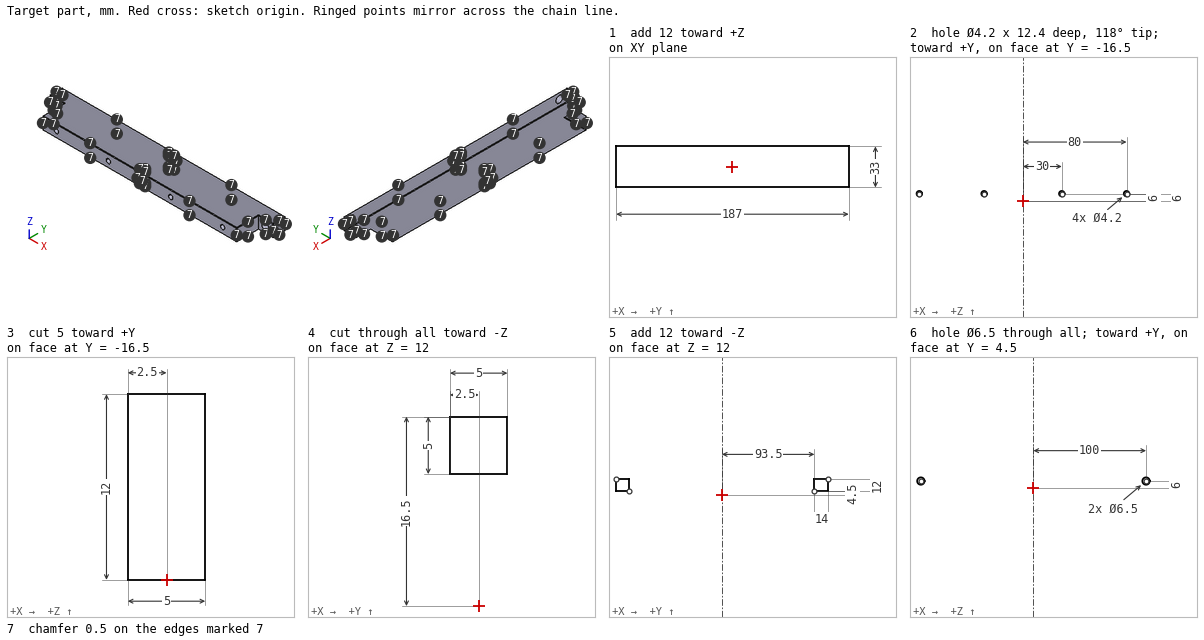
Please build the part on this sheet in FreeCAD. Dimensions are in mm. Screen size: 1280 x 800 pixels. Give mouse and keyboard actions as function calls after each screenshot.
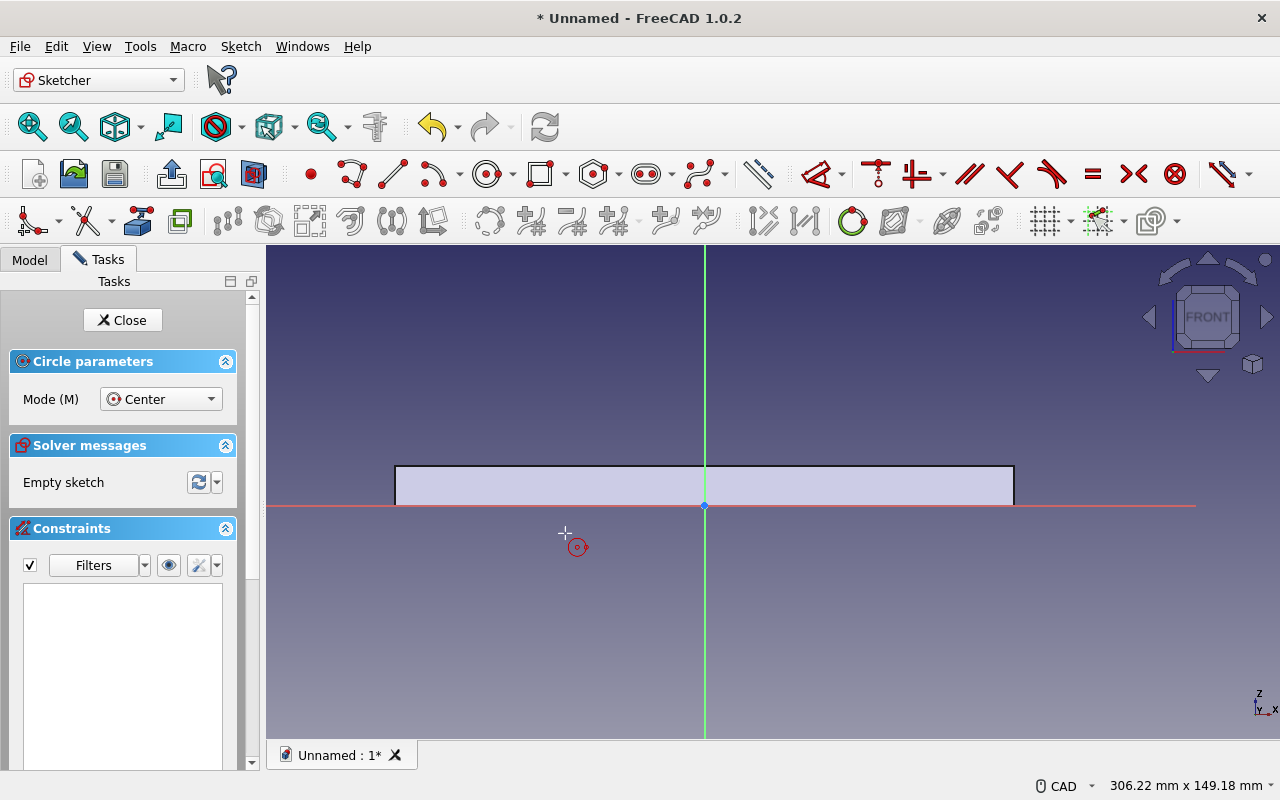
scroll(969, 486, up, 6)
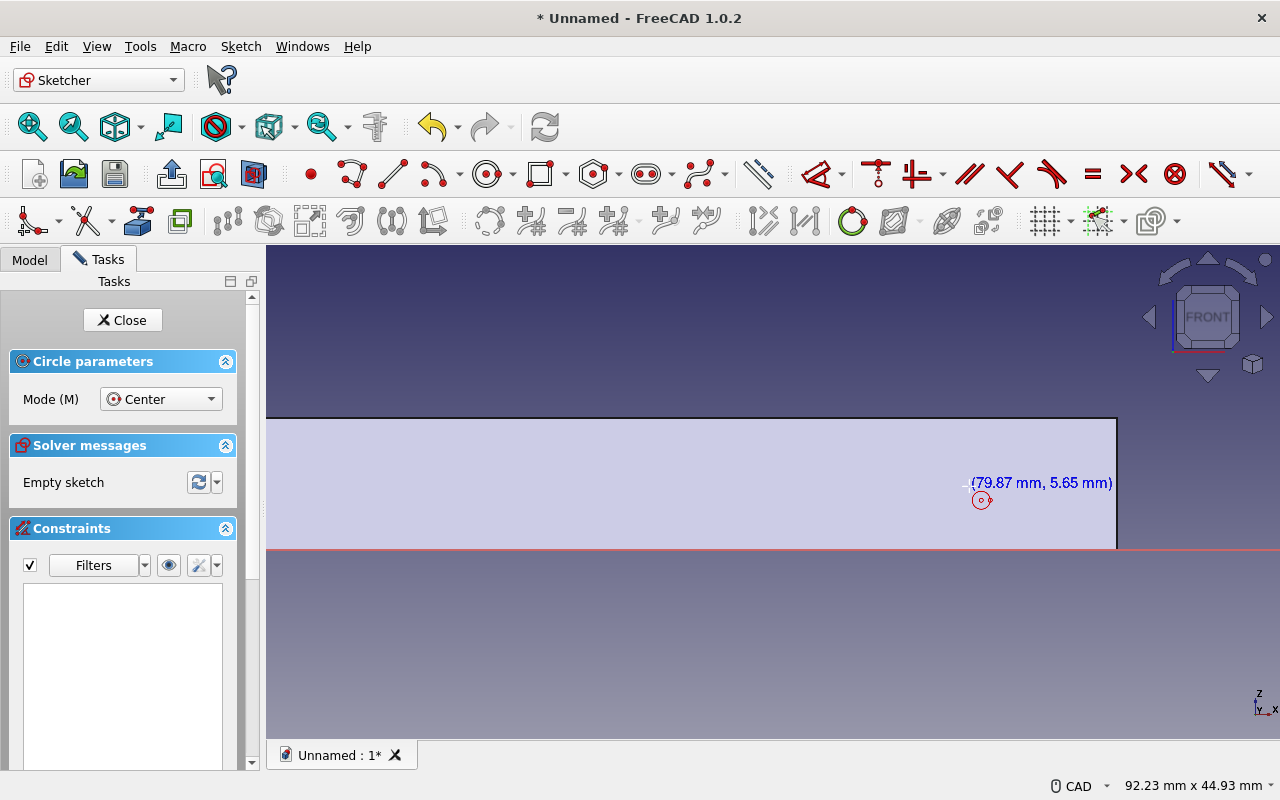
click(969, 484)
click(985, 468)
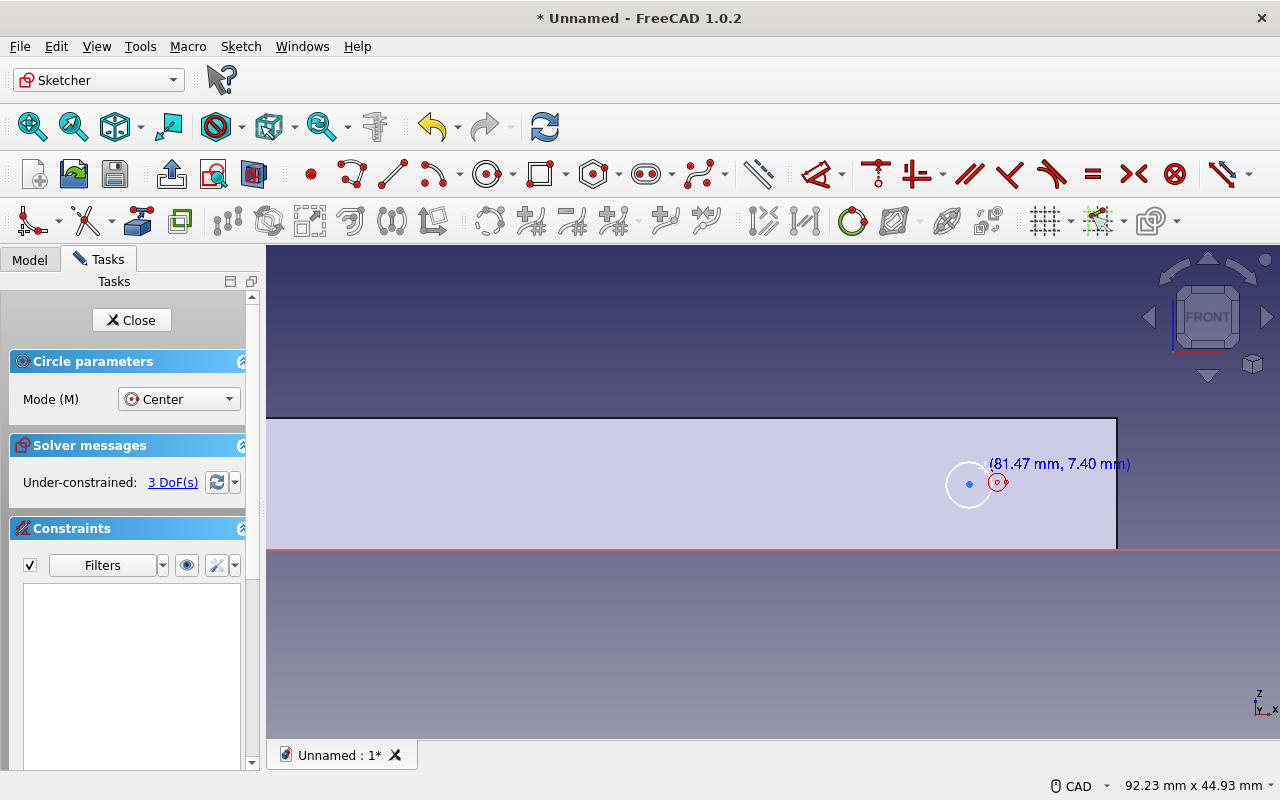
click(419, 484)
click(435, 468)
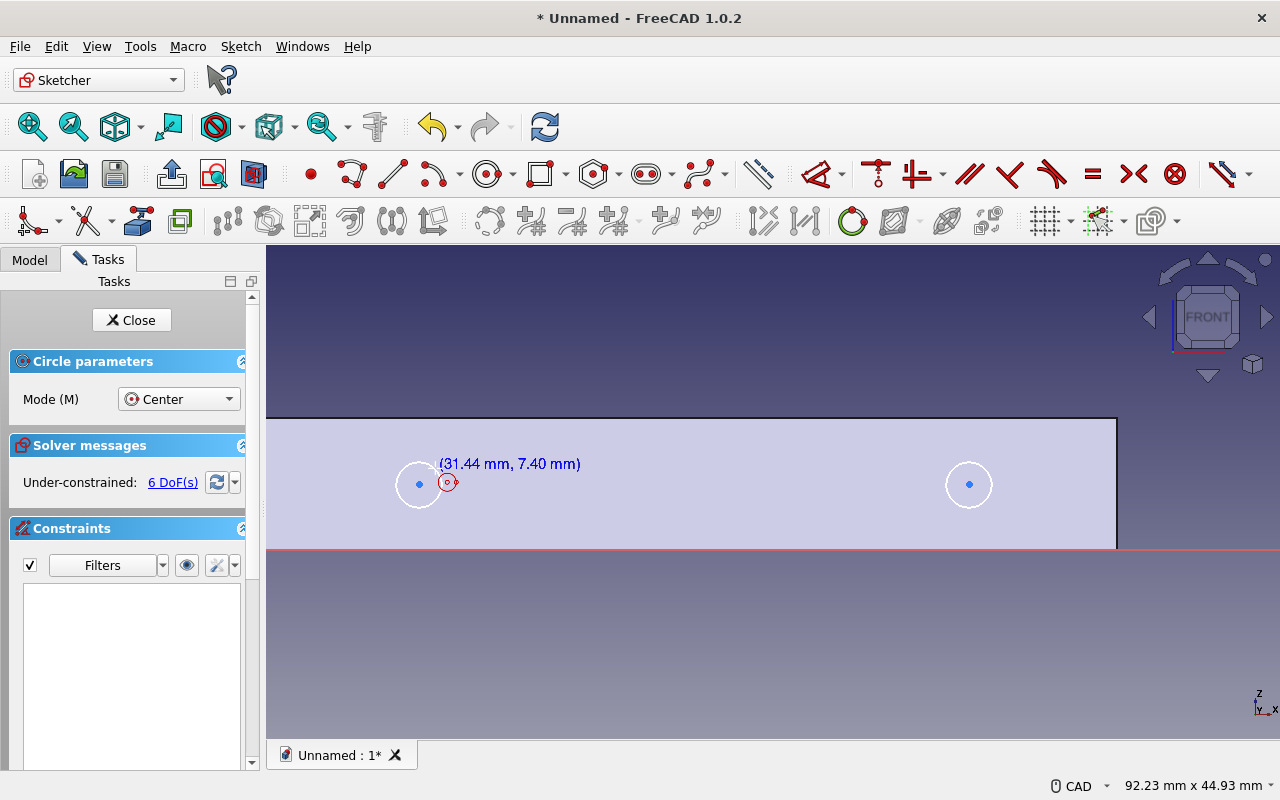
scroll(970, 486, down, 6)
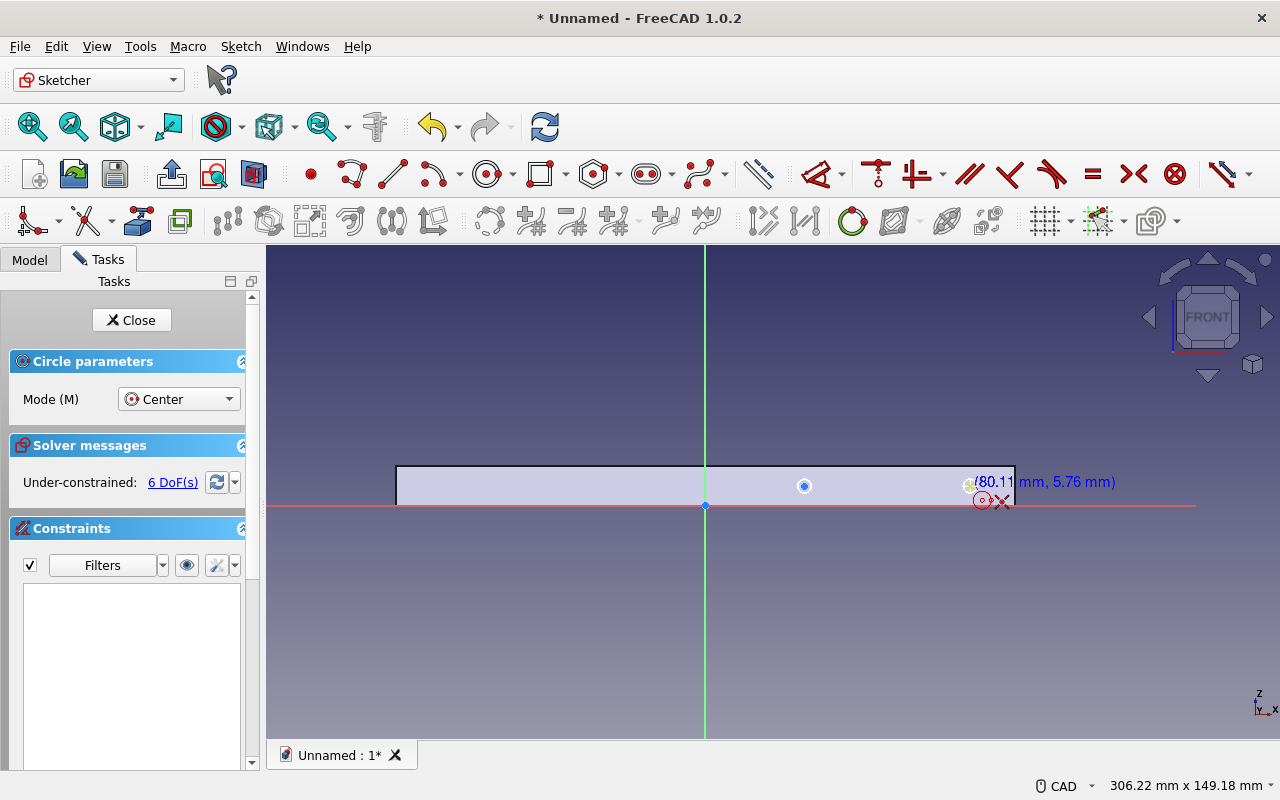
scroll(606, 486, up, 6)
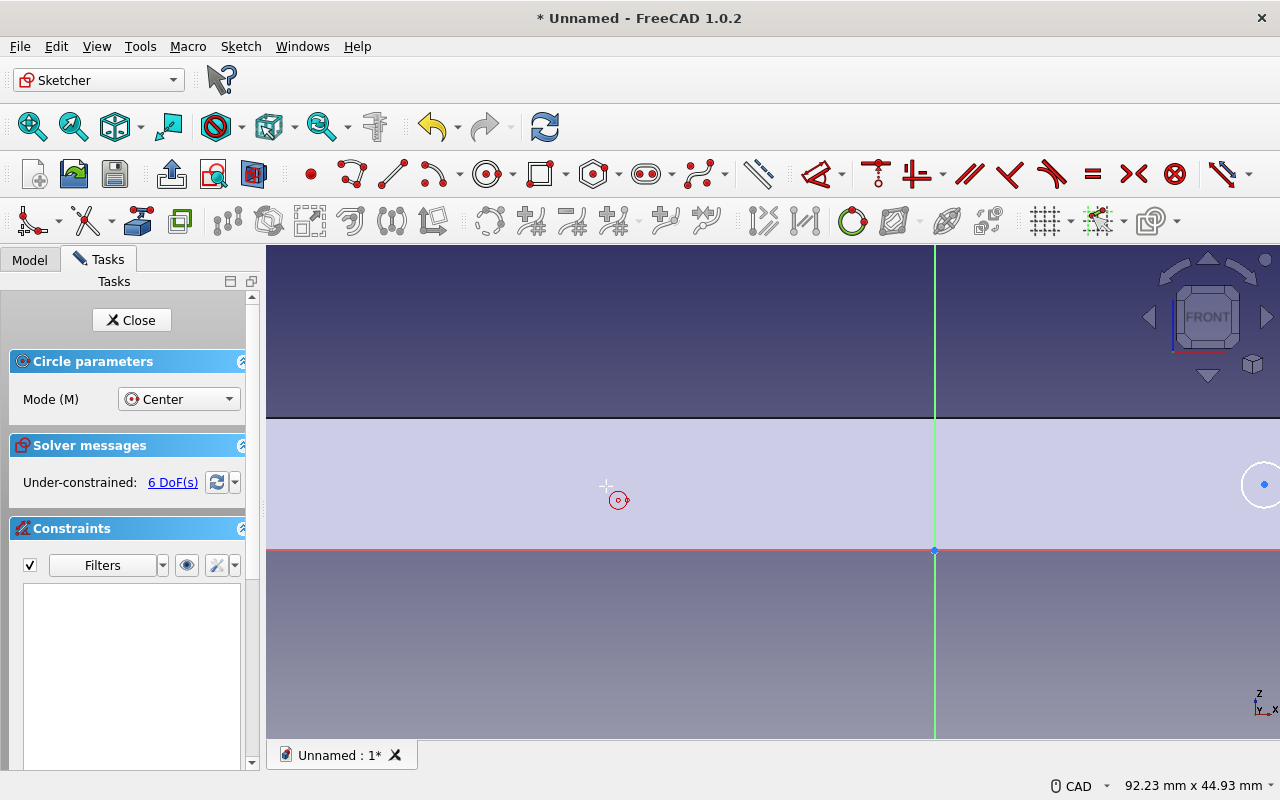
click(605, 484)
click(621, 468)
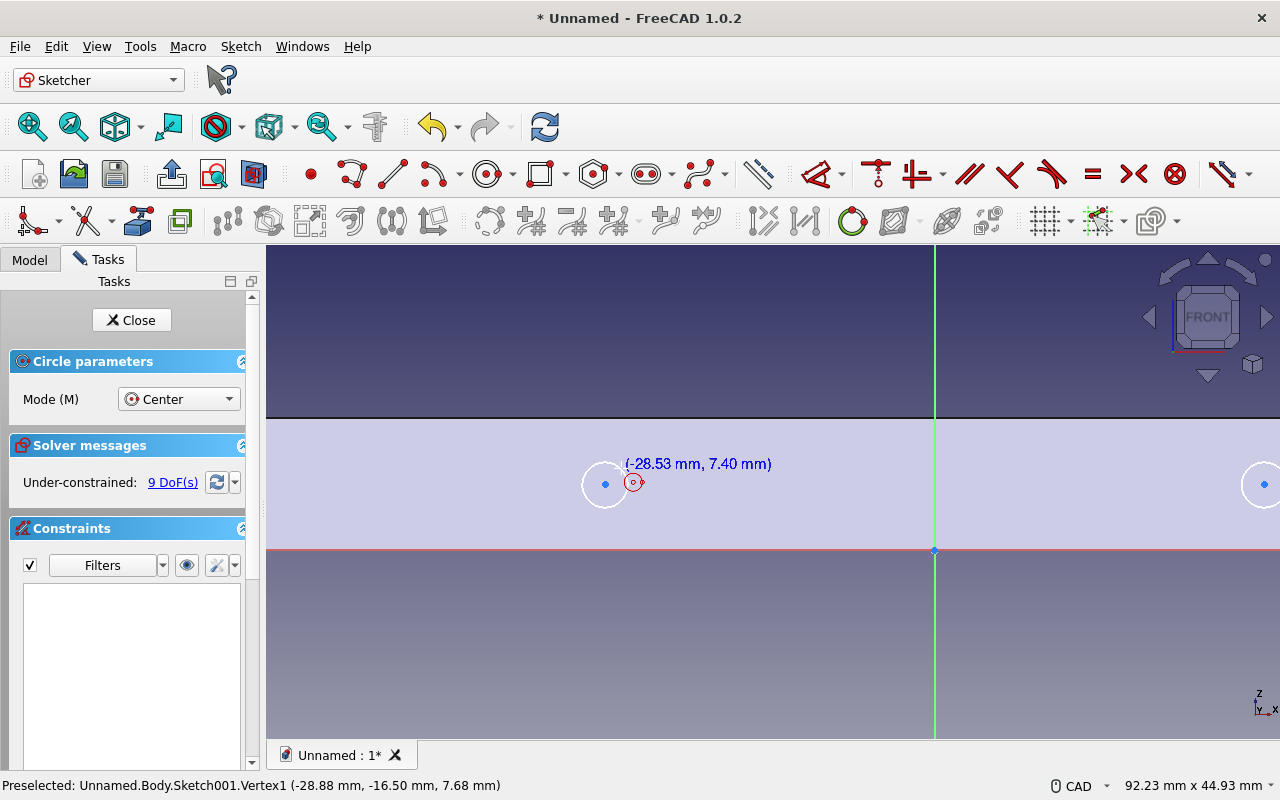
scroll(605, 486, down, 6)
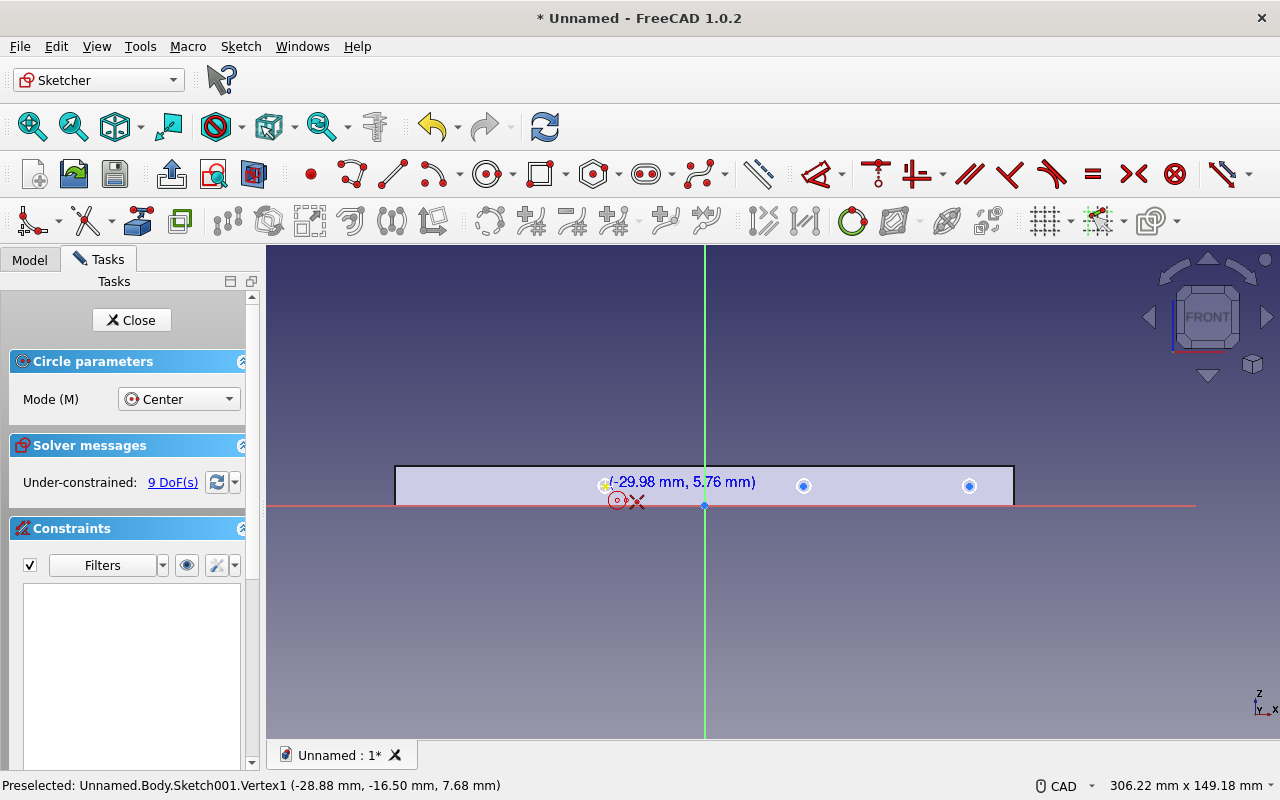
scroll(440, 486, up, 6)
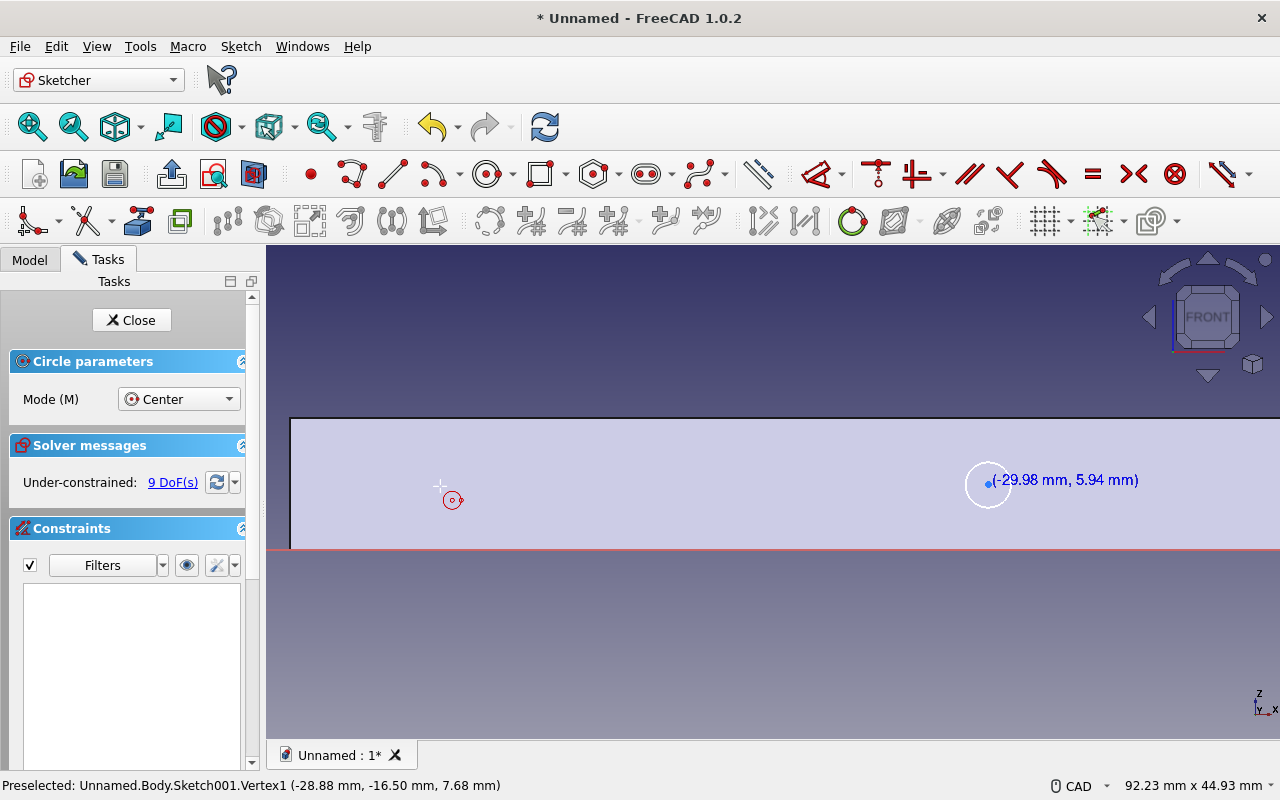
click(438, 484)
click(455, 468)
key(Escape)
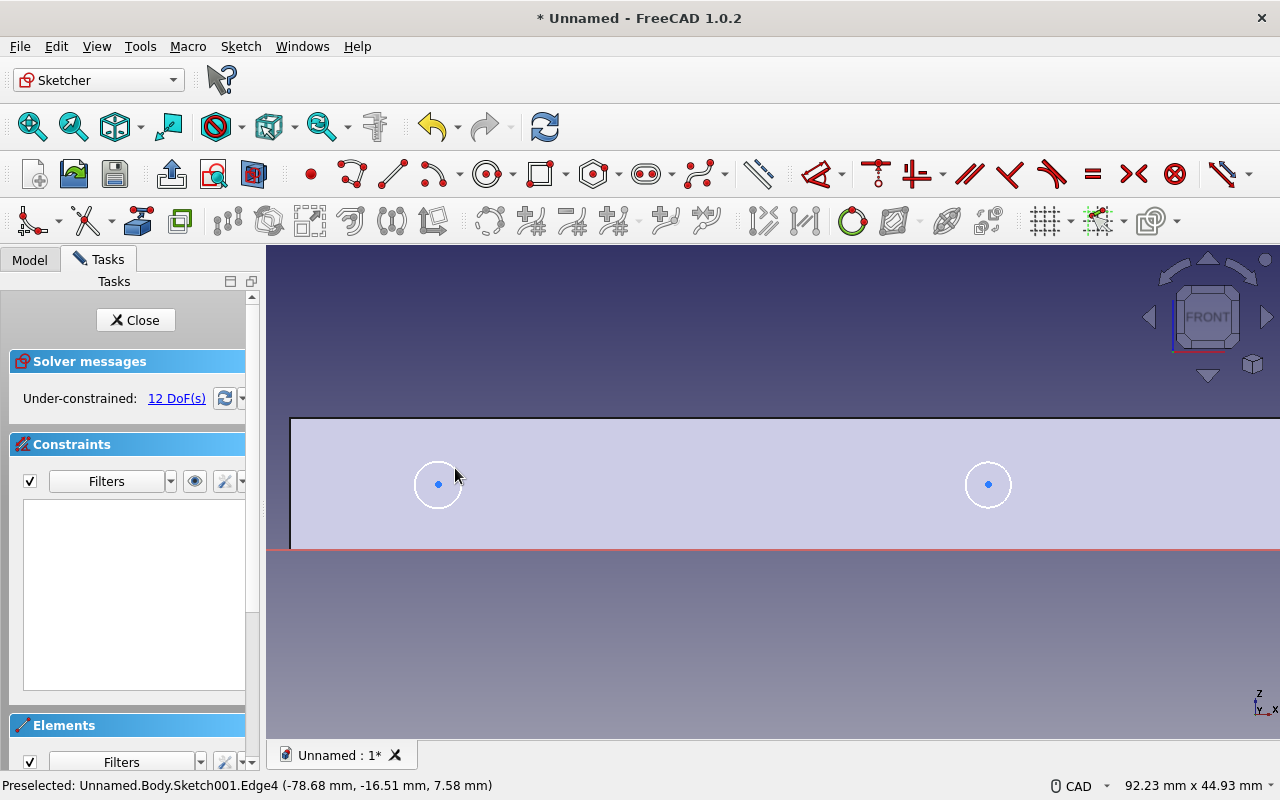
scroll(440, 486, down, 6)